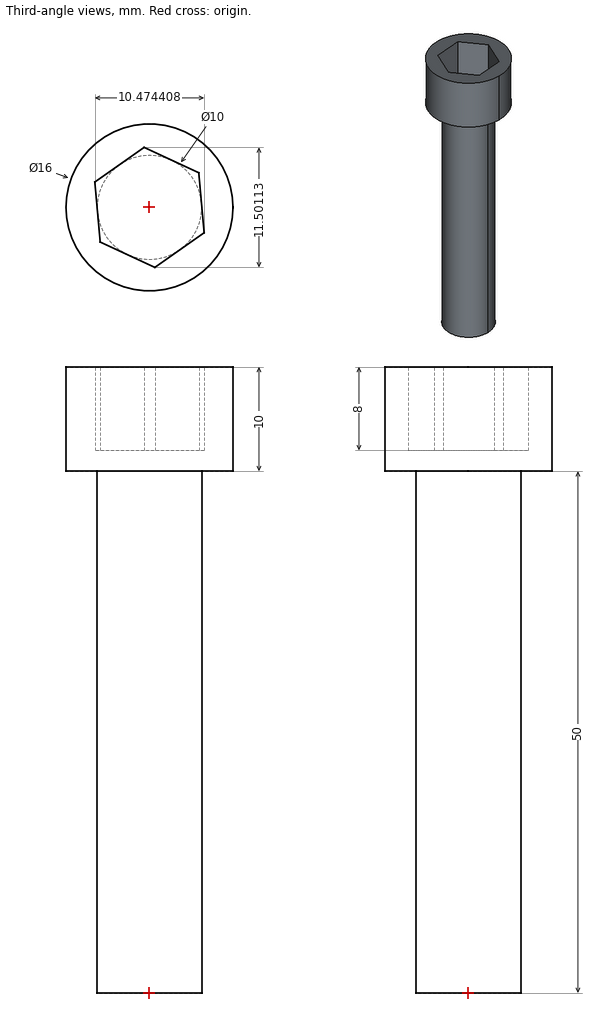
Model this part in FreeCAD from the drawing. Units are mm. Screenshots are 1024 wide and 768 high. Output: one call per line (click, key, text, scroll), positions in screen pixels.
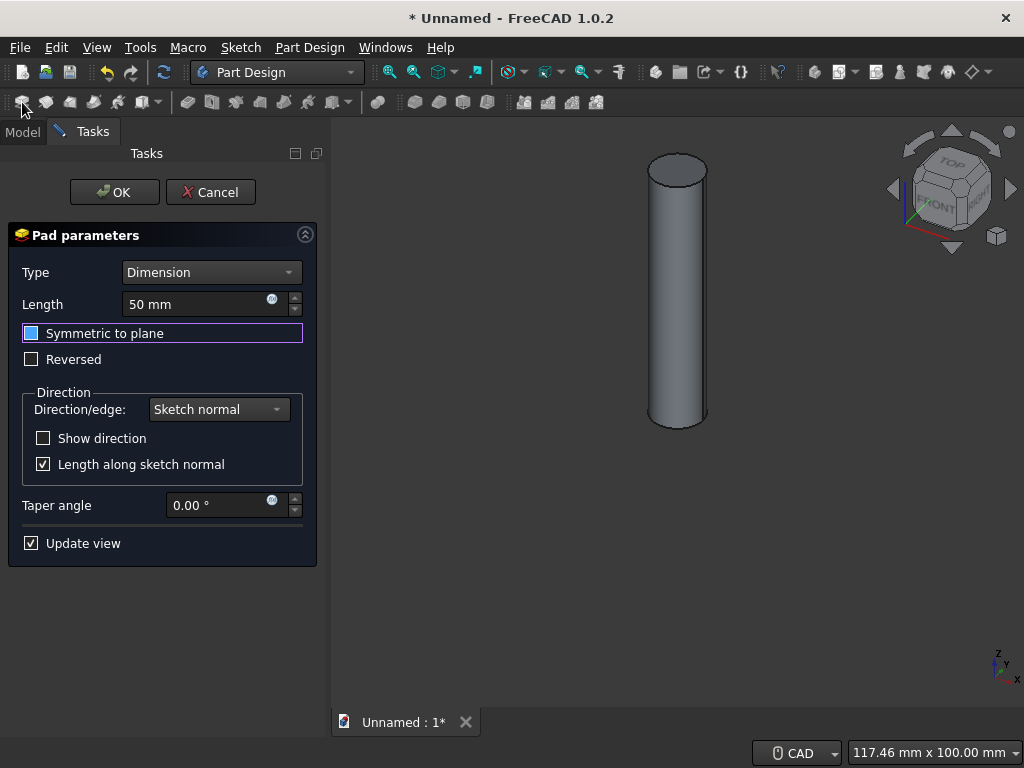
click(115, 192)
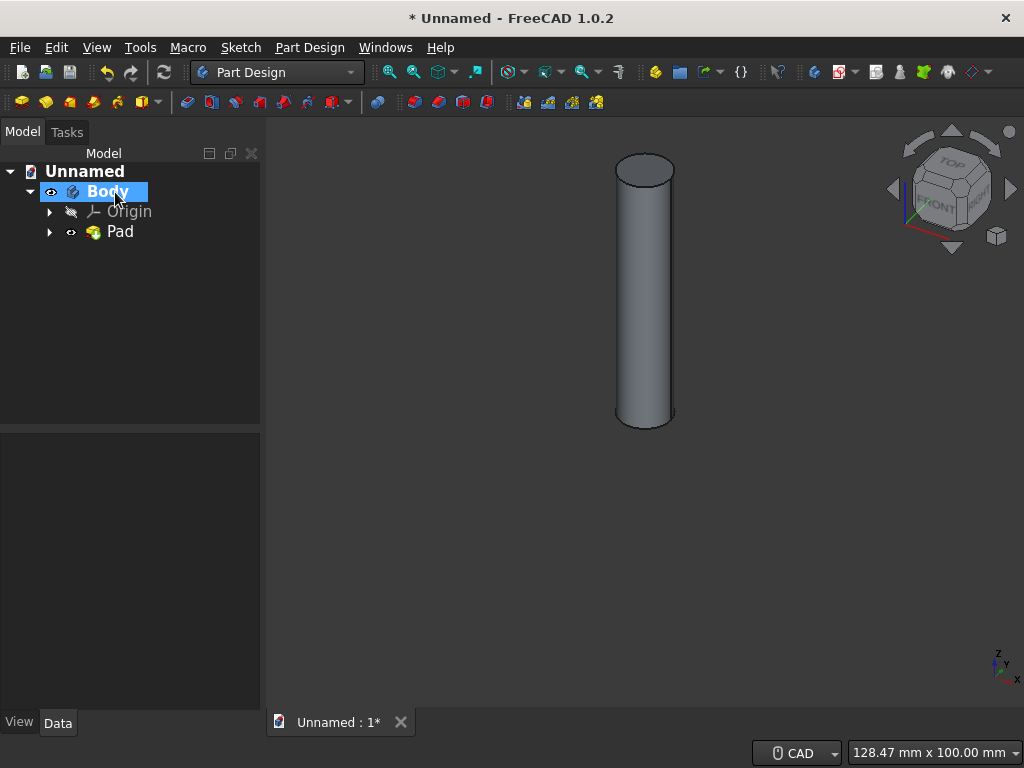
click(645, 169)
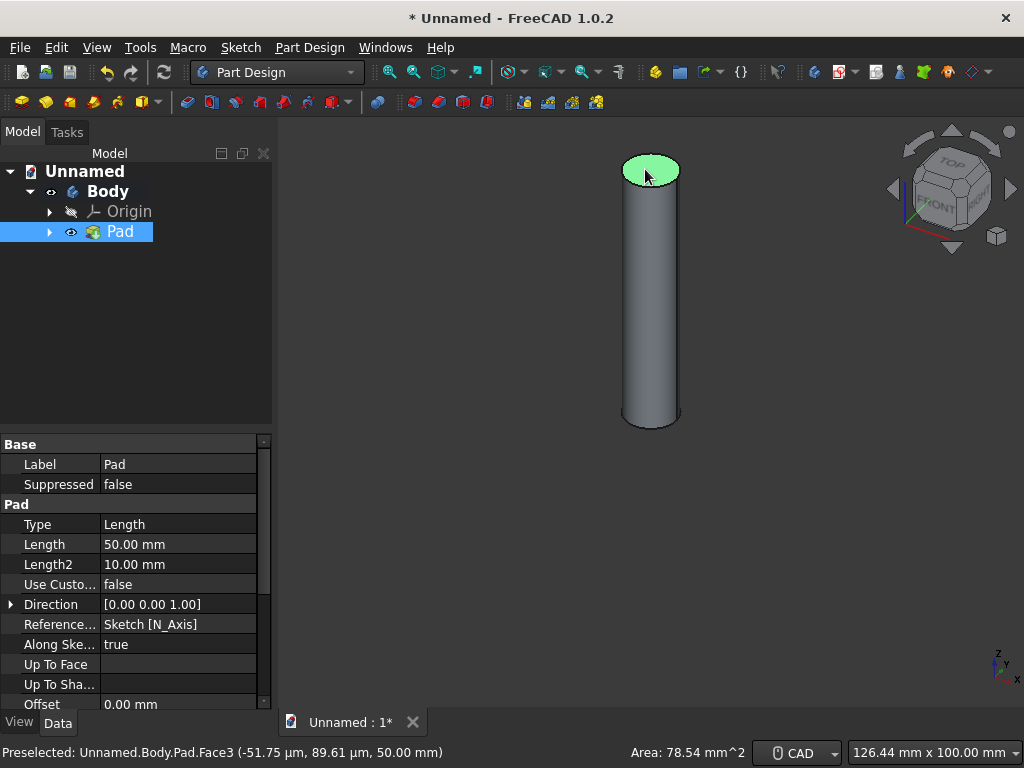
click(840, 72)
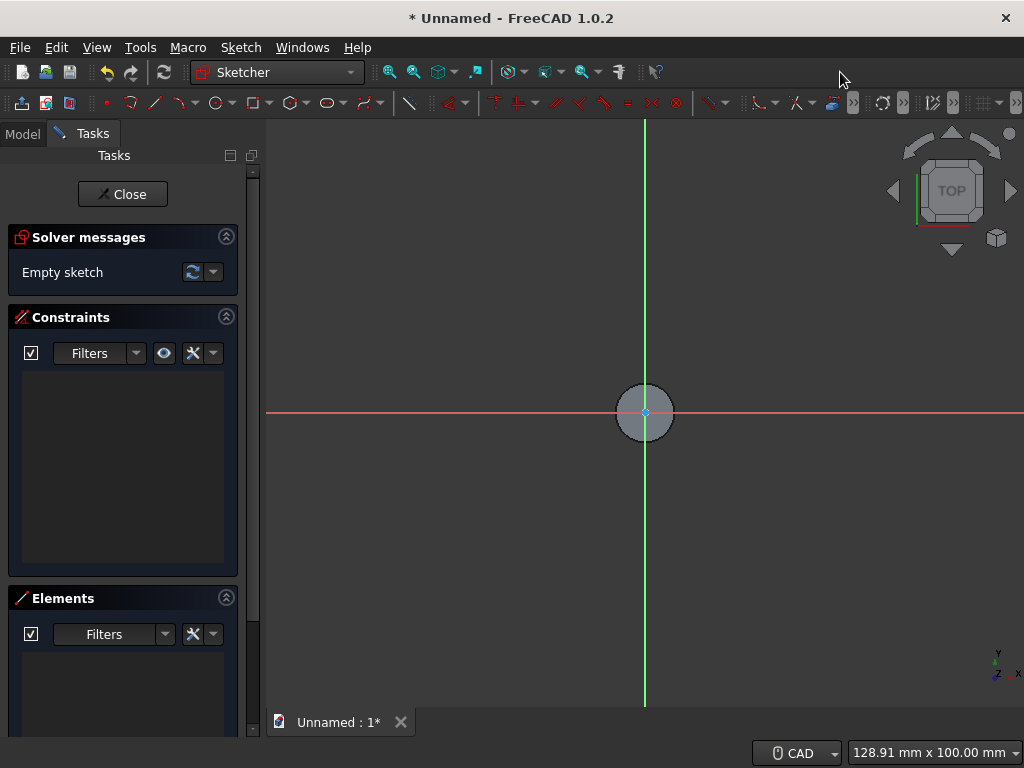
scroll(667, 413, up, 7)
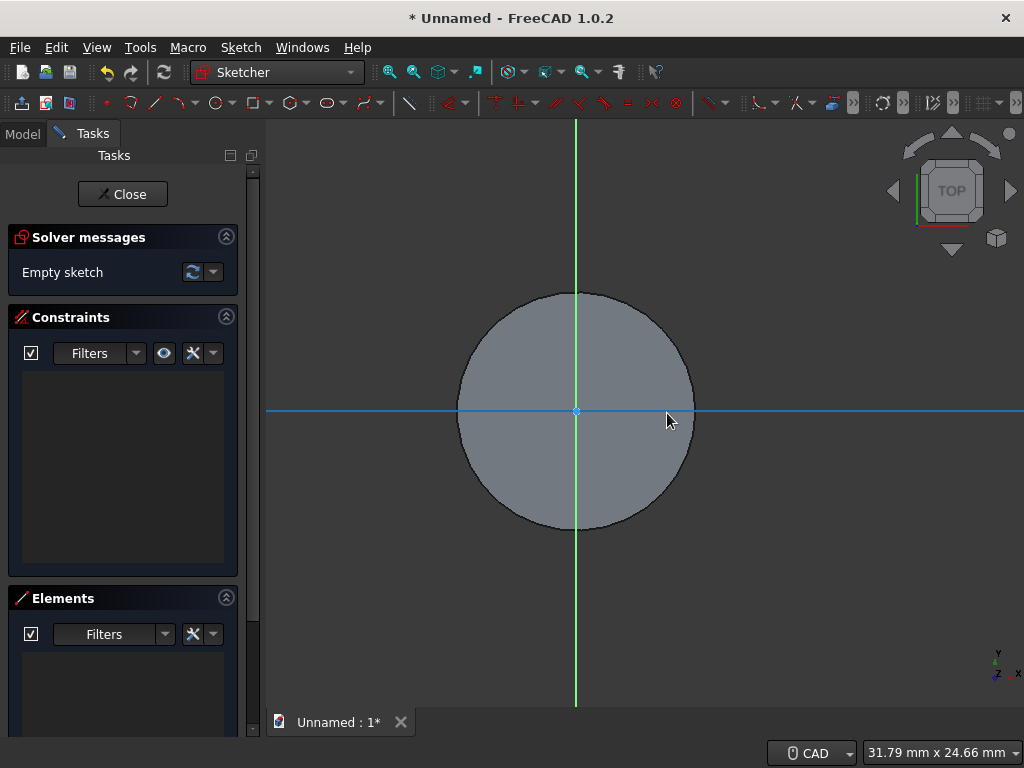
key(g)
key(c)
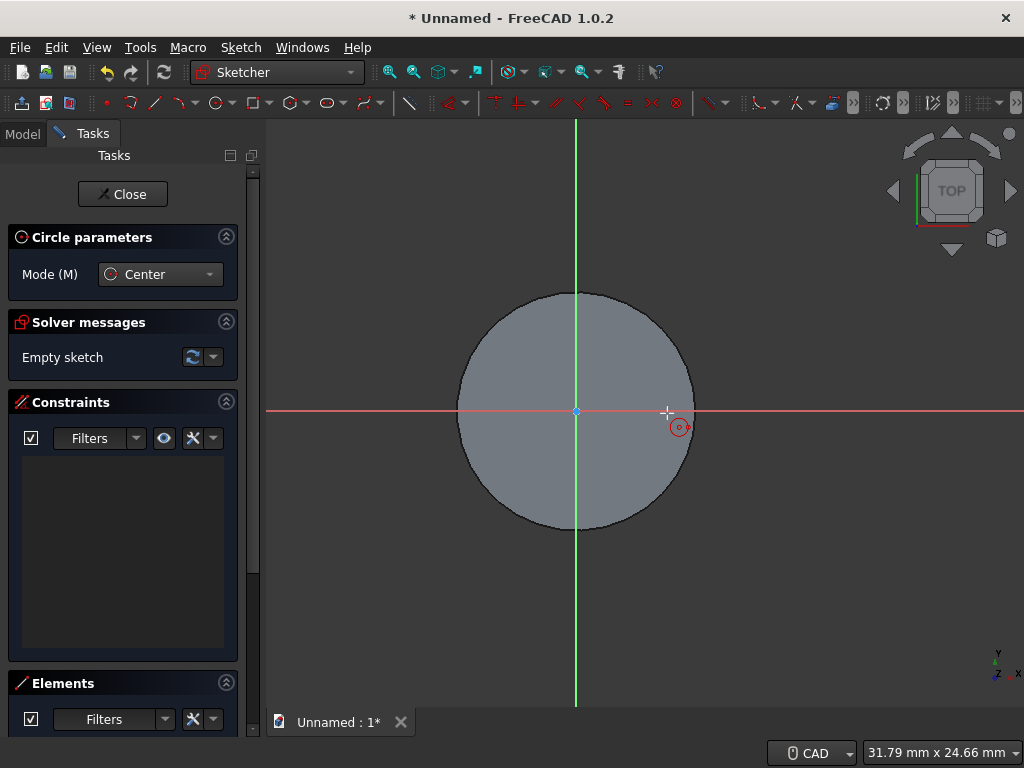
click(576, 411)
click(711, 277)
key(Escape)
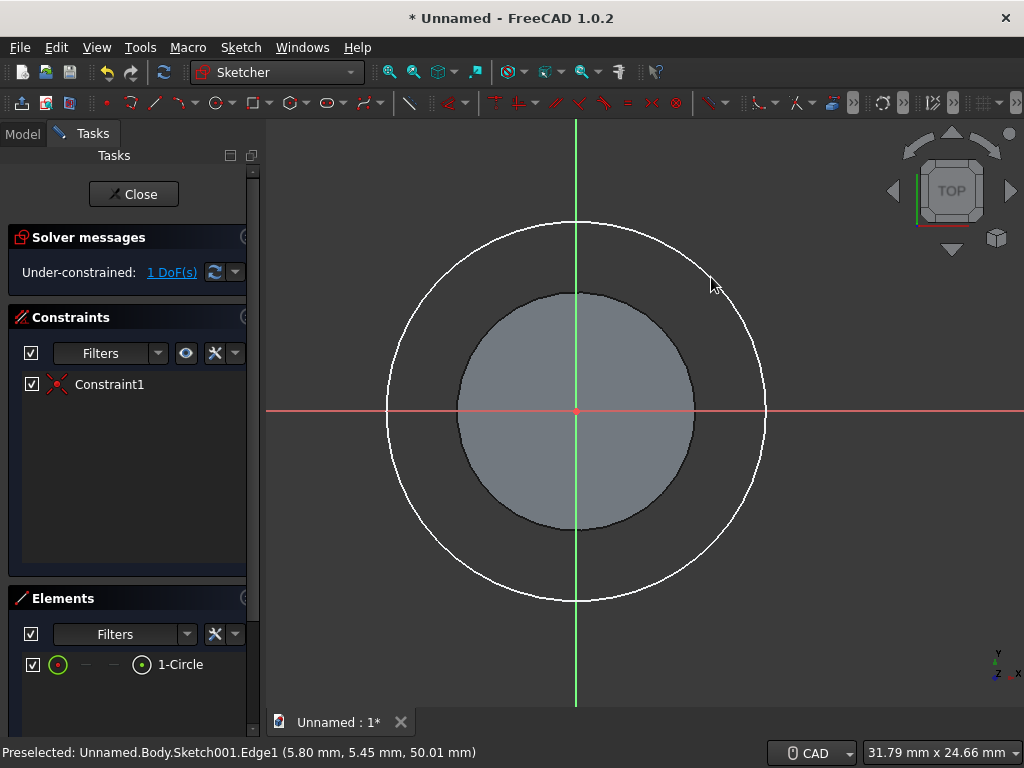
click(710, 277)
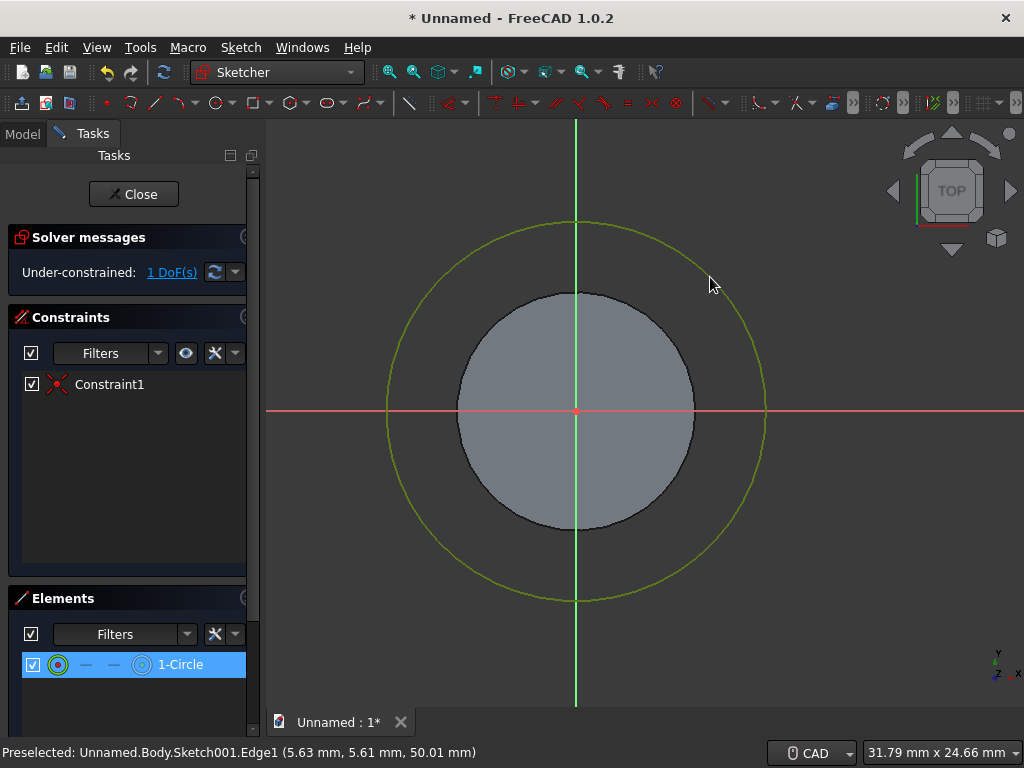
key(k)
key(o)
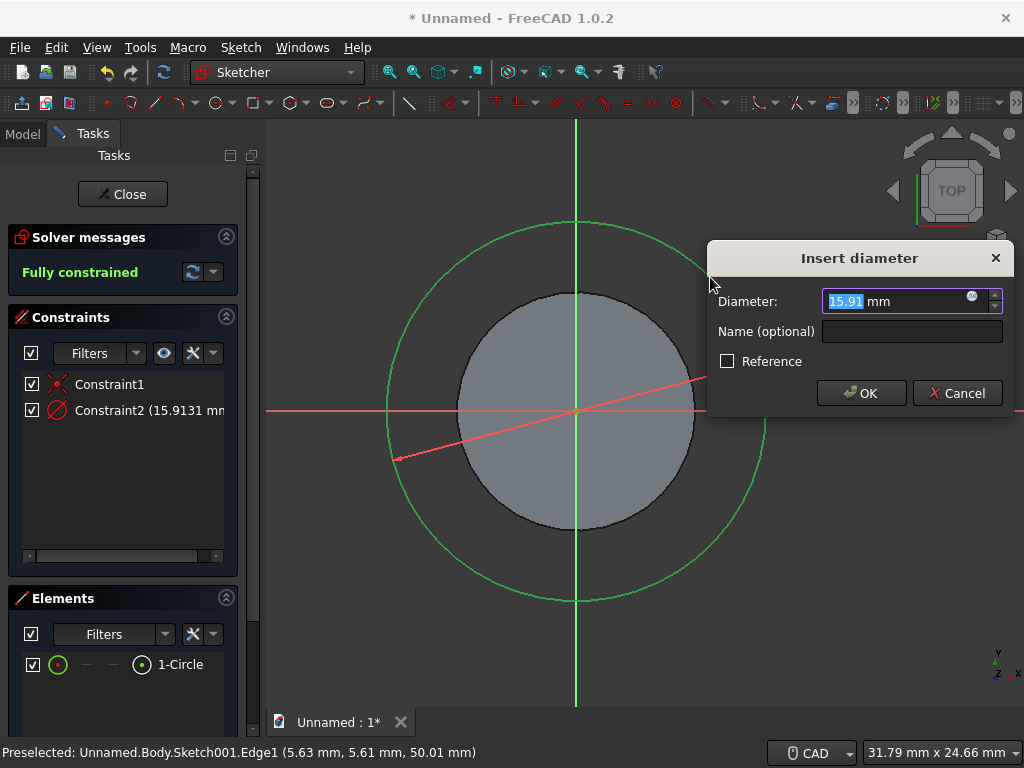
text(16)
key(Return)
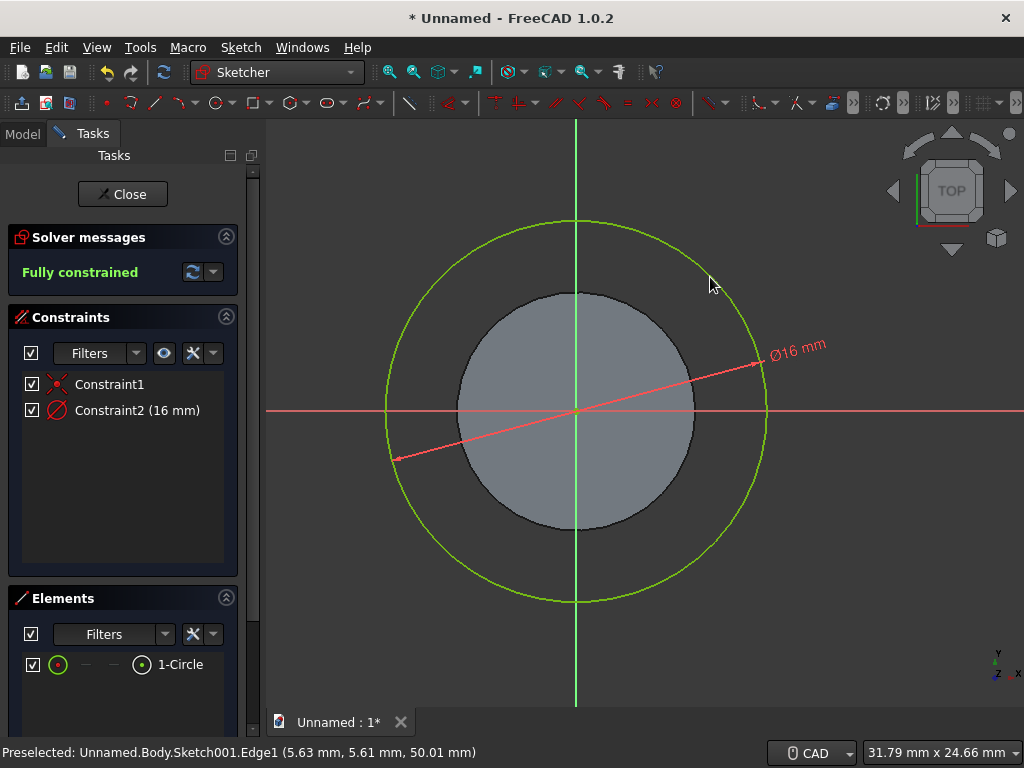
click(123, 194)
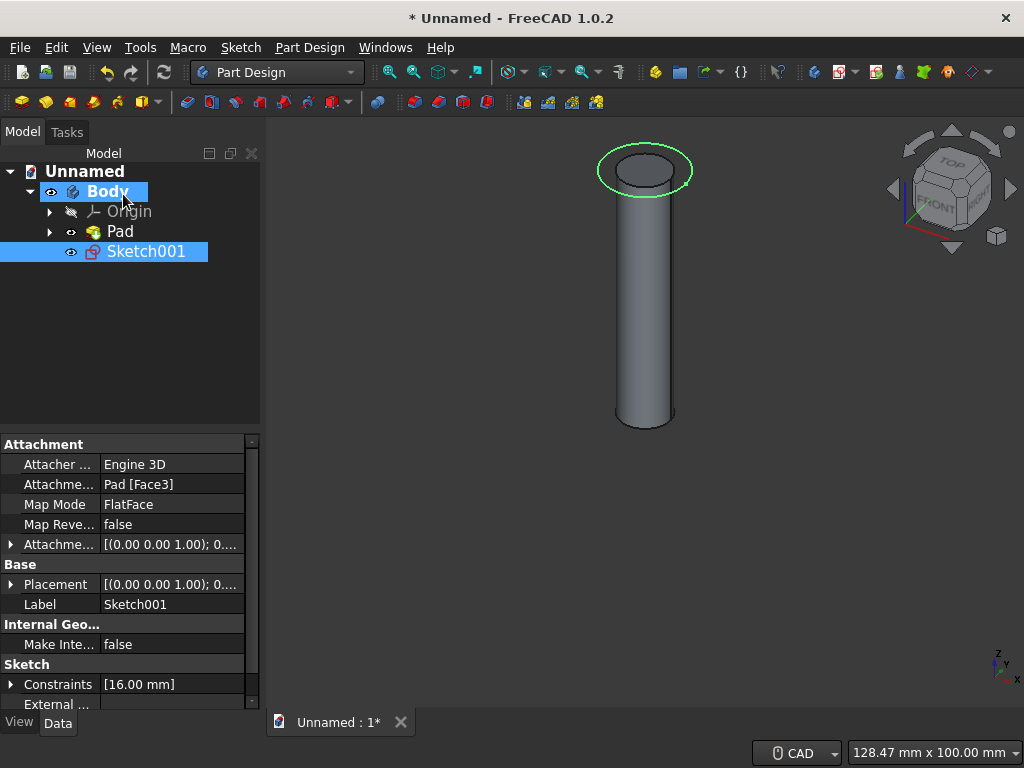
click(22, 102)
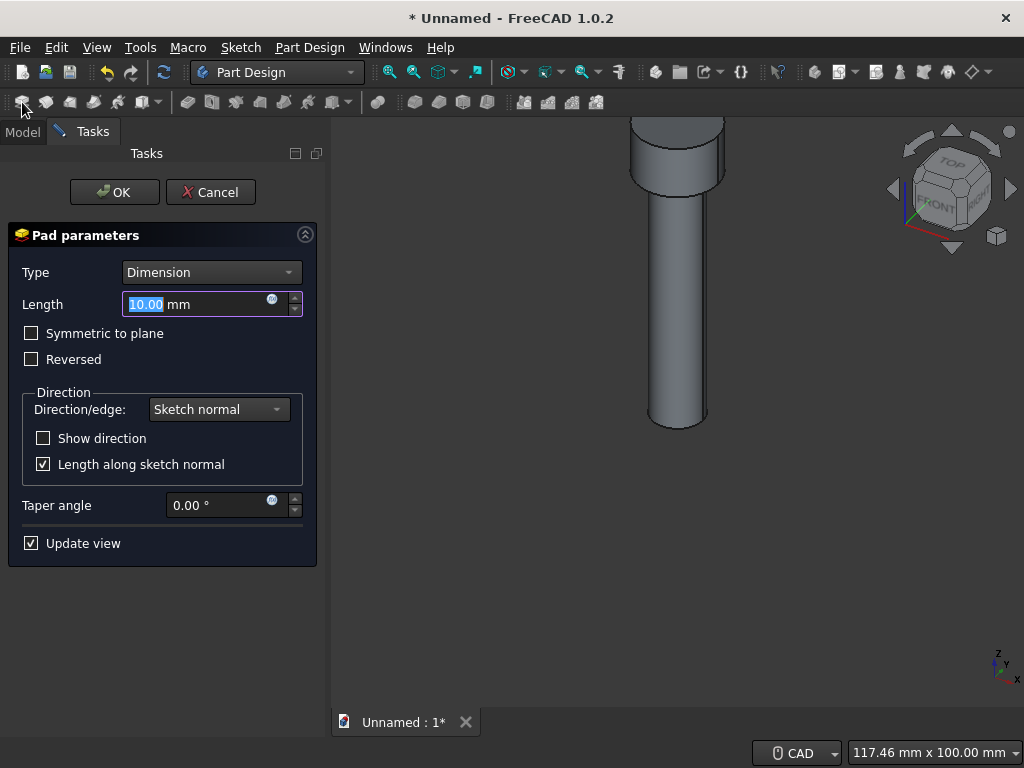
text(10)
key(Tab)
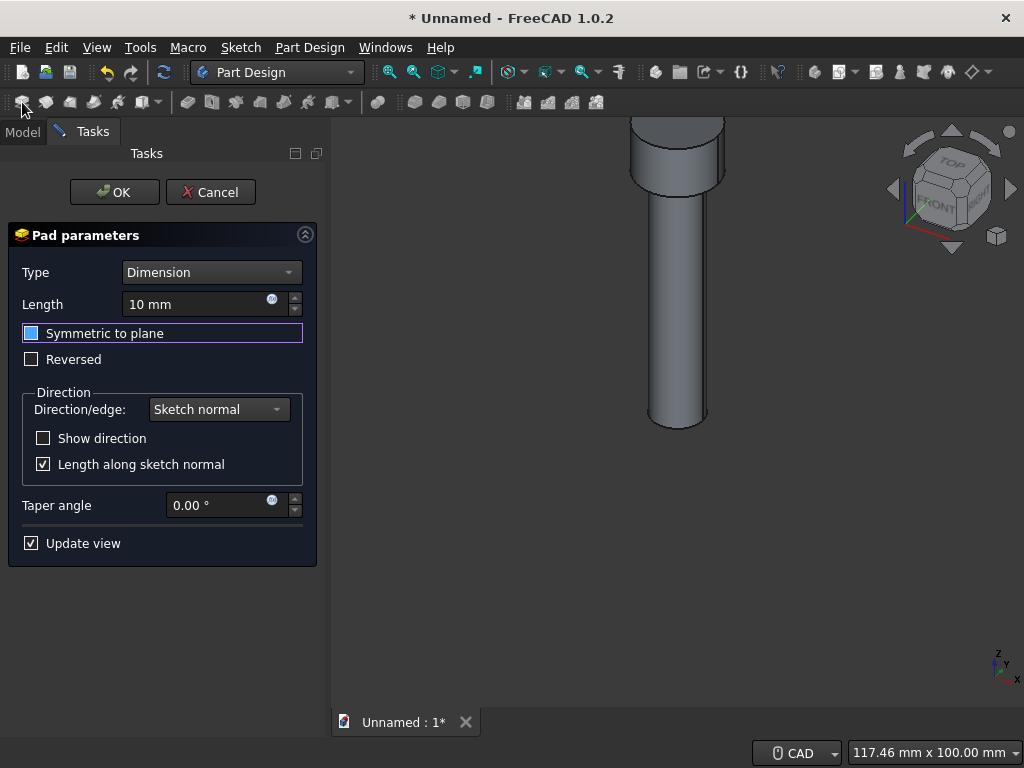
click(115, 192)